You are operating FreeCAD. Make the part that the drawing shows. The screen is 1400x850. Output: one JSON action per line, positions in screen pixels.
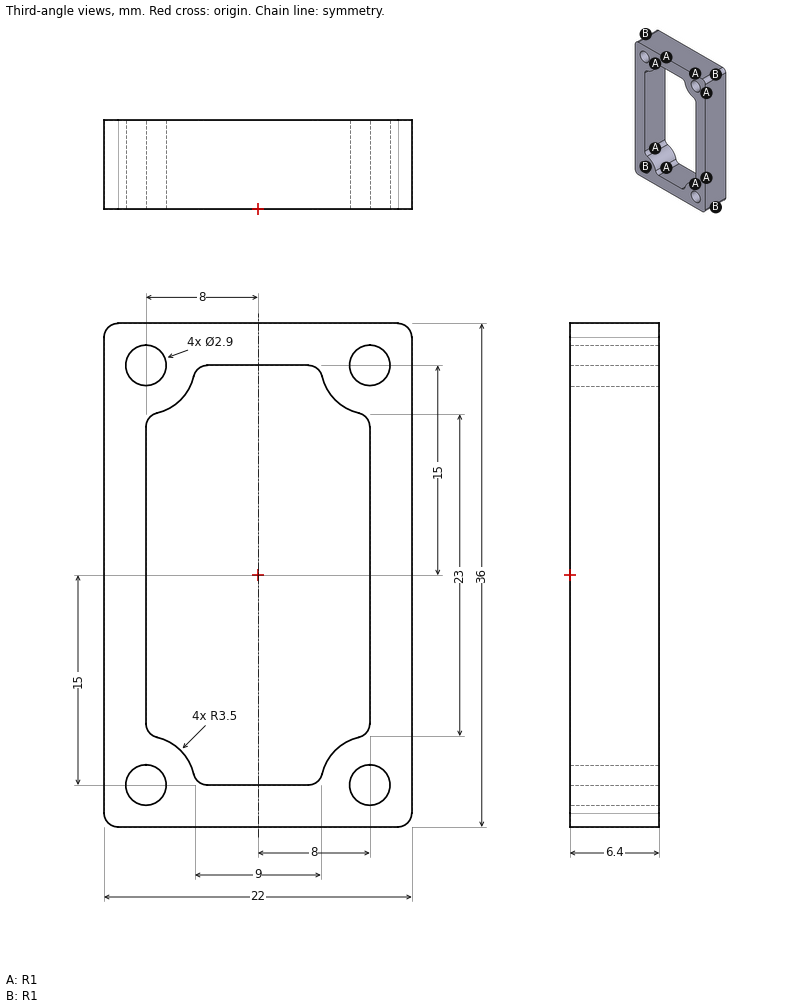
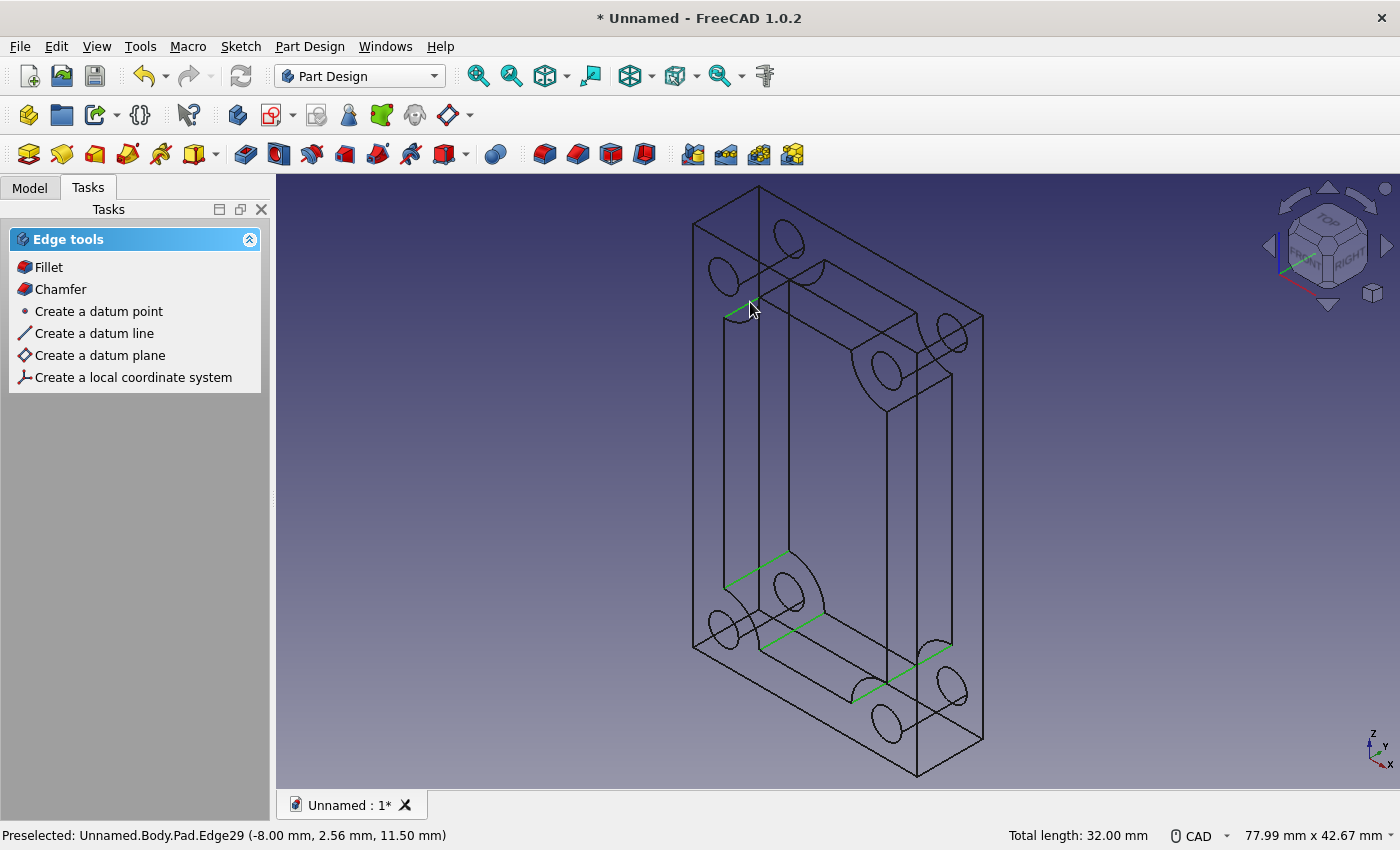
{"action": "left_click", "coordinate": [799, 274], "text": "ctrl"}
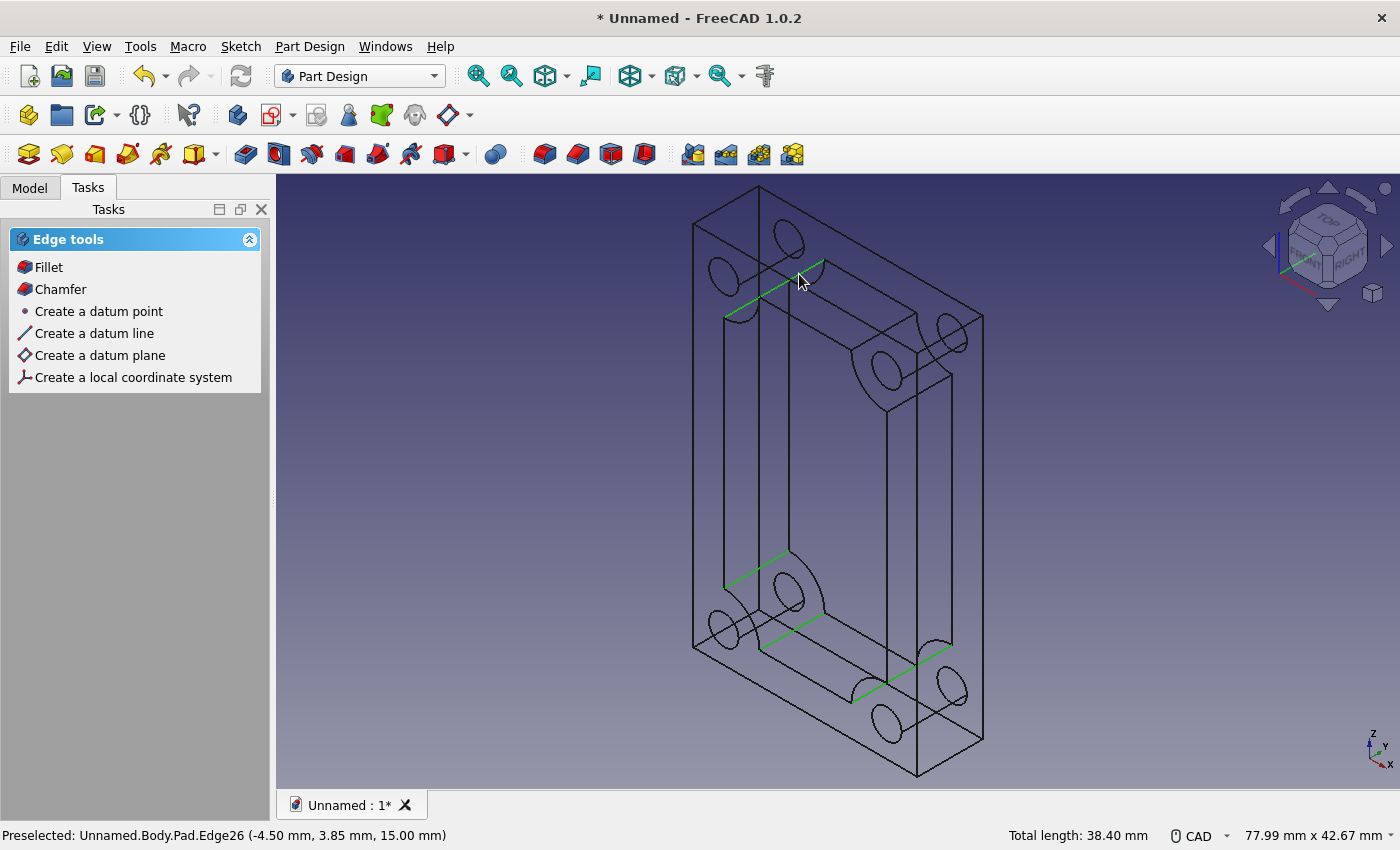
{"action": "left_click", "coordinate": [890, 327], "text": "ctrl"}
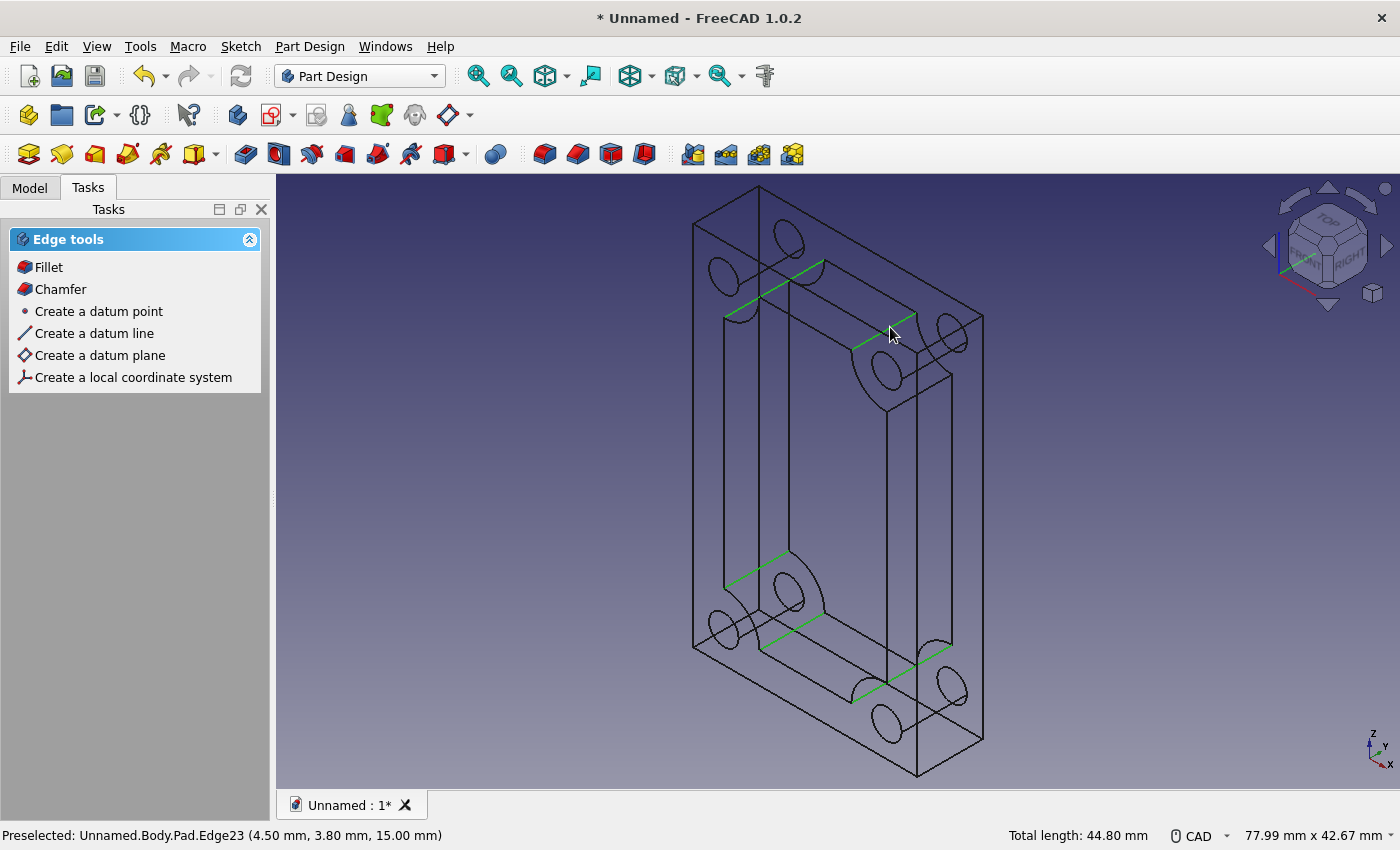
{"action": "left_click", "coordinate": [926, 388], "text": "ctrl"}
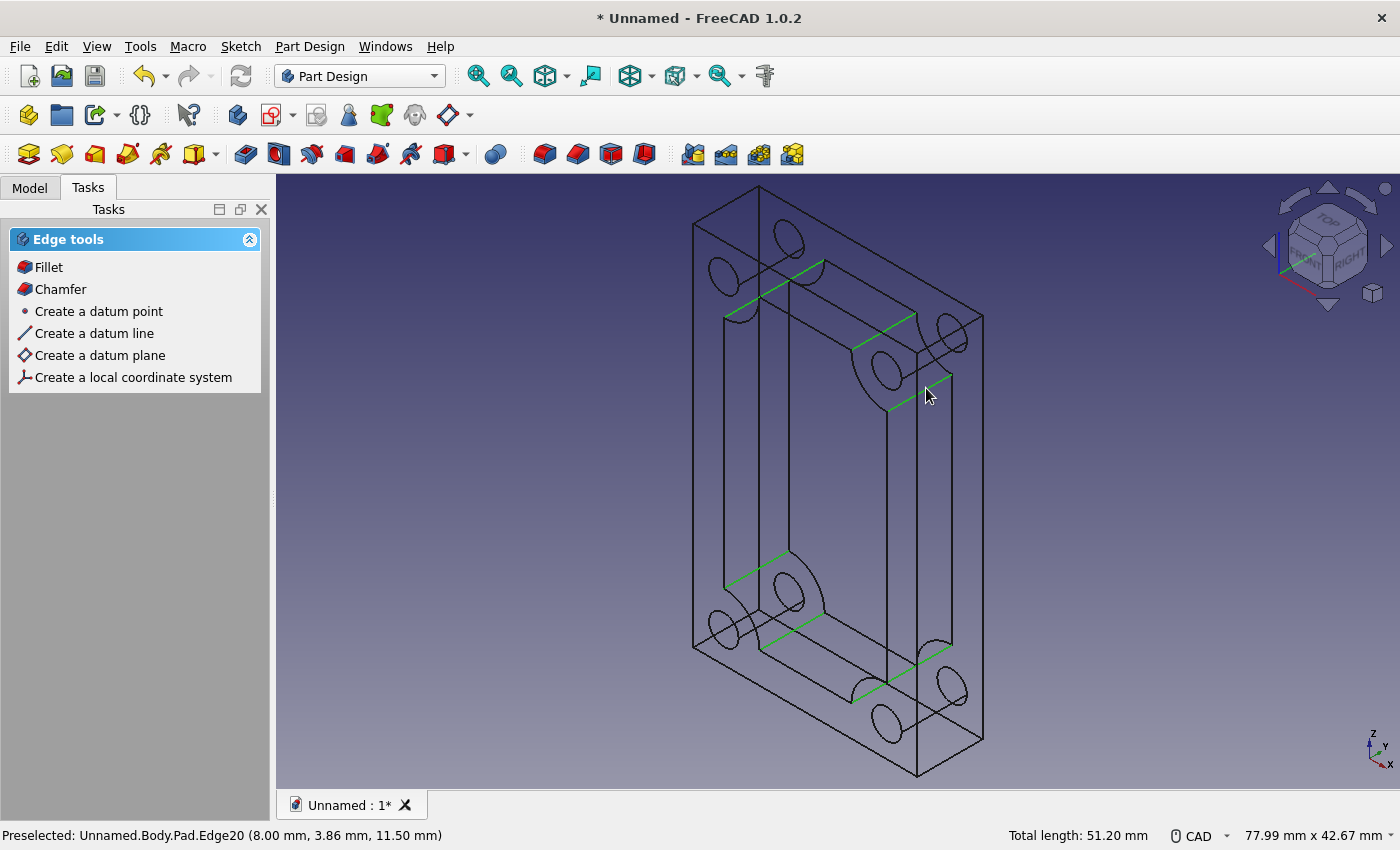
{"action": "key", "text": "v 1"}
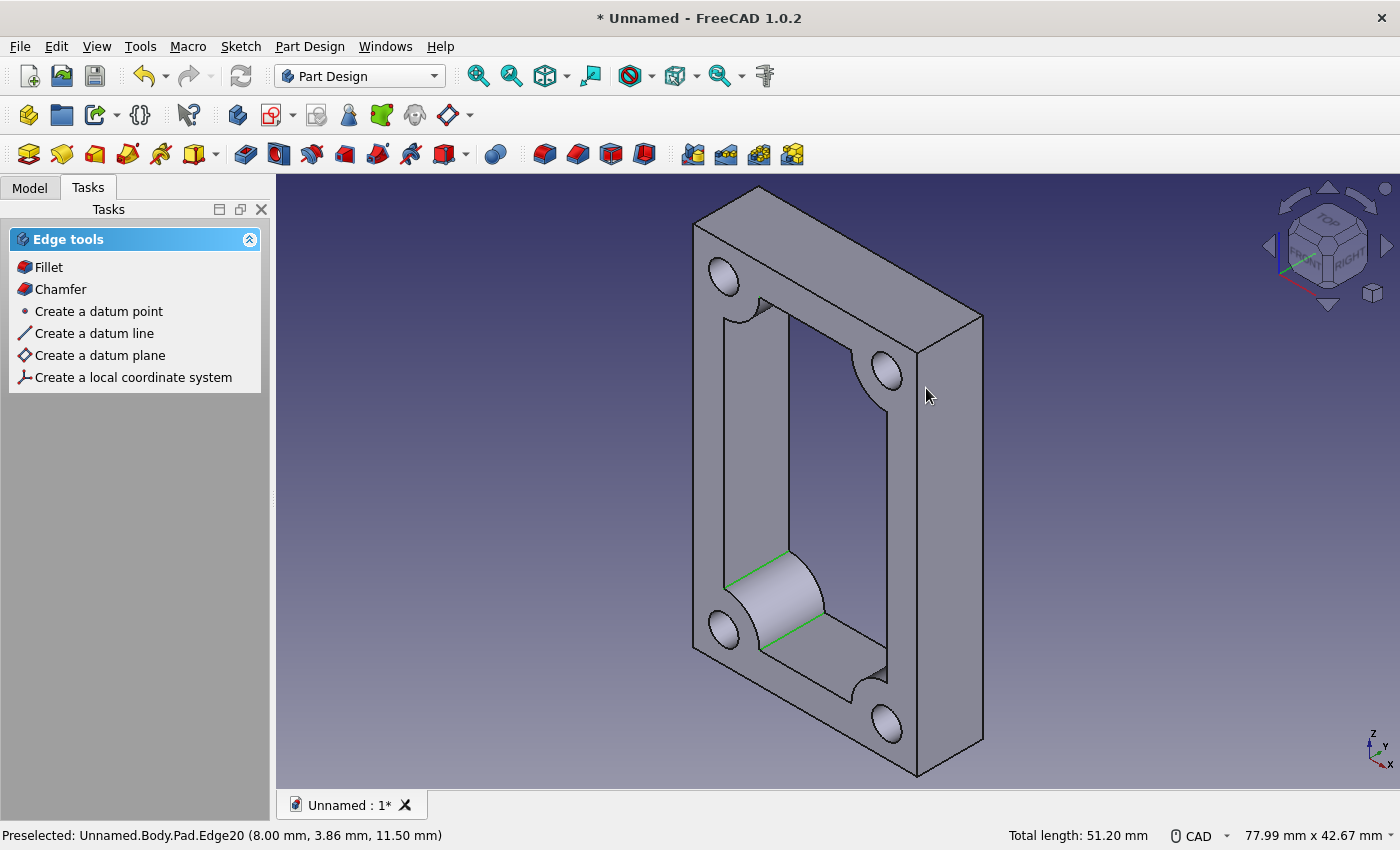
{"action": "left_click", "coordinate": [545, 154]}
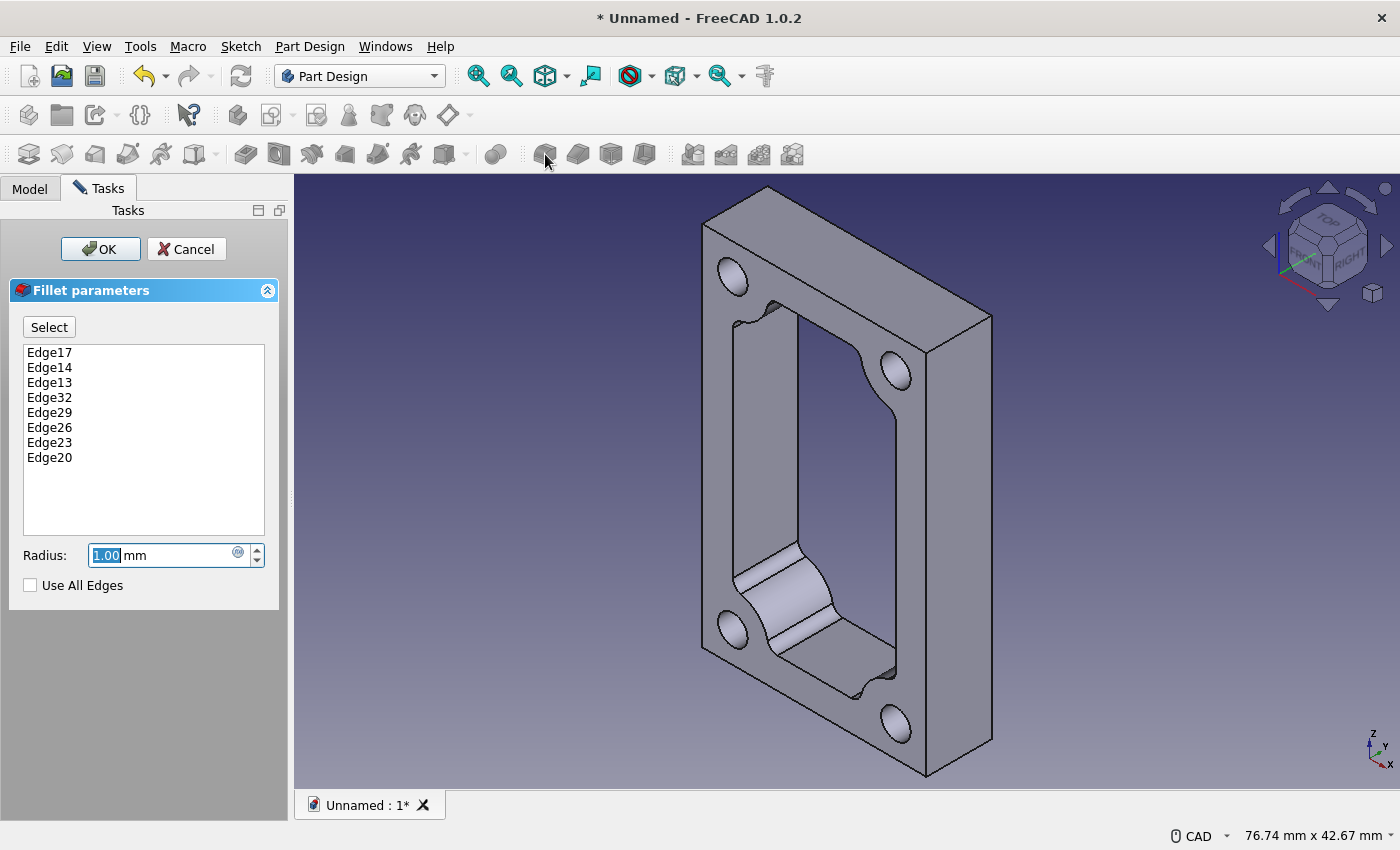
{"action": "type", "text": "1"}
{"action": "key", "text": "Tab"}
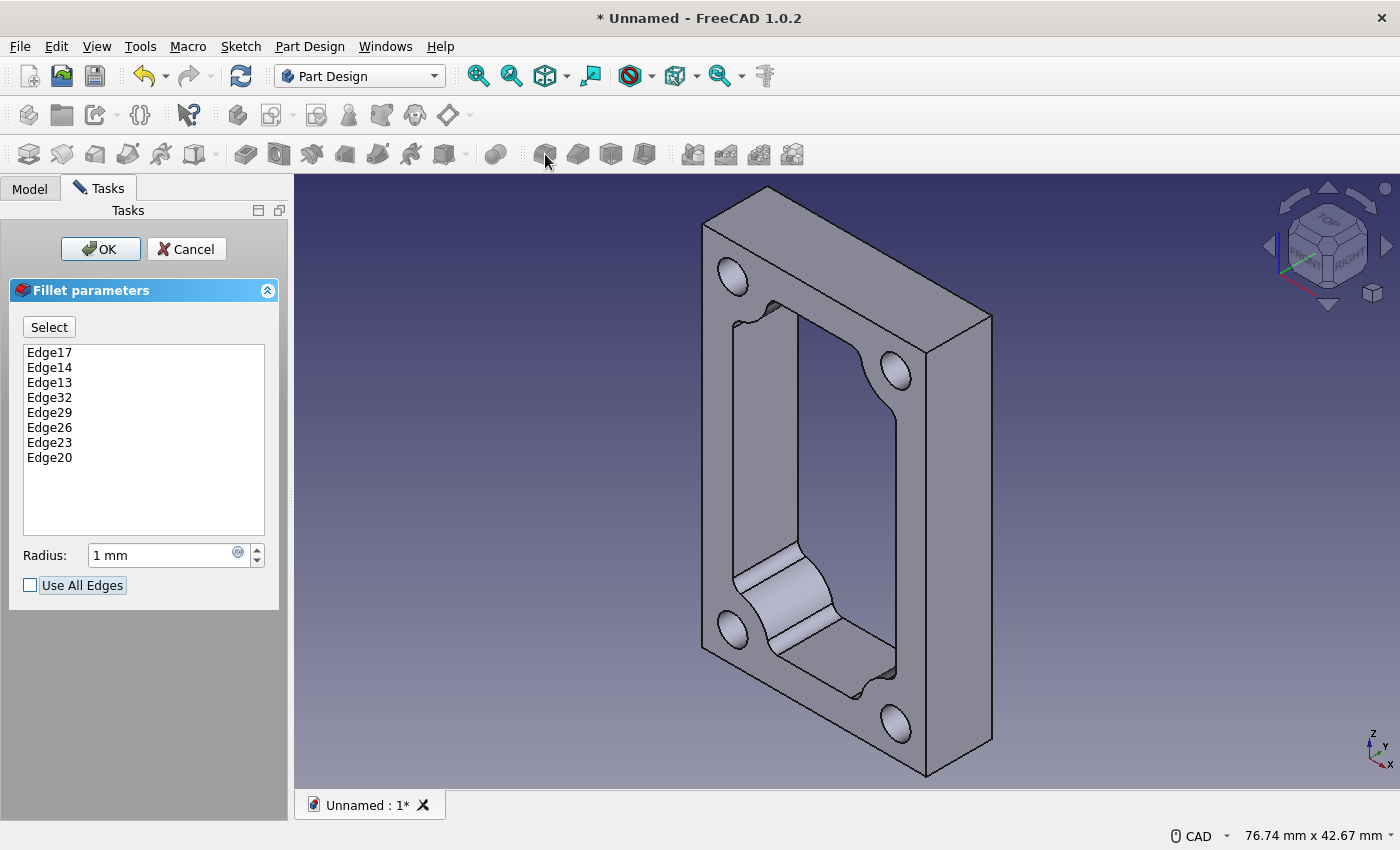
{"action": "left_click", "coordinate": [101, 249]}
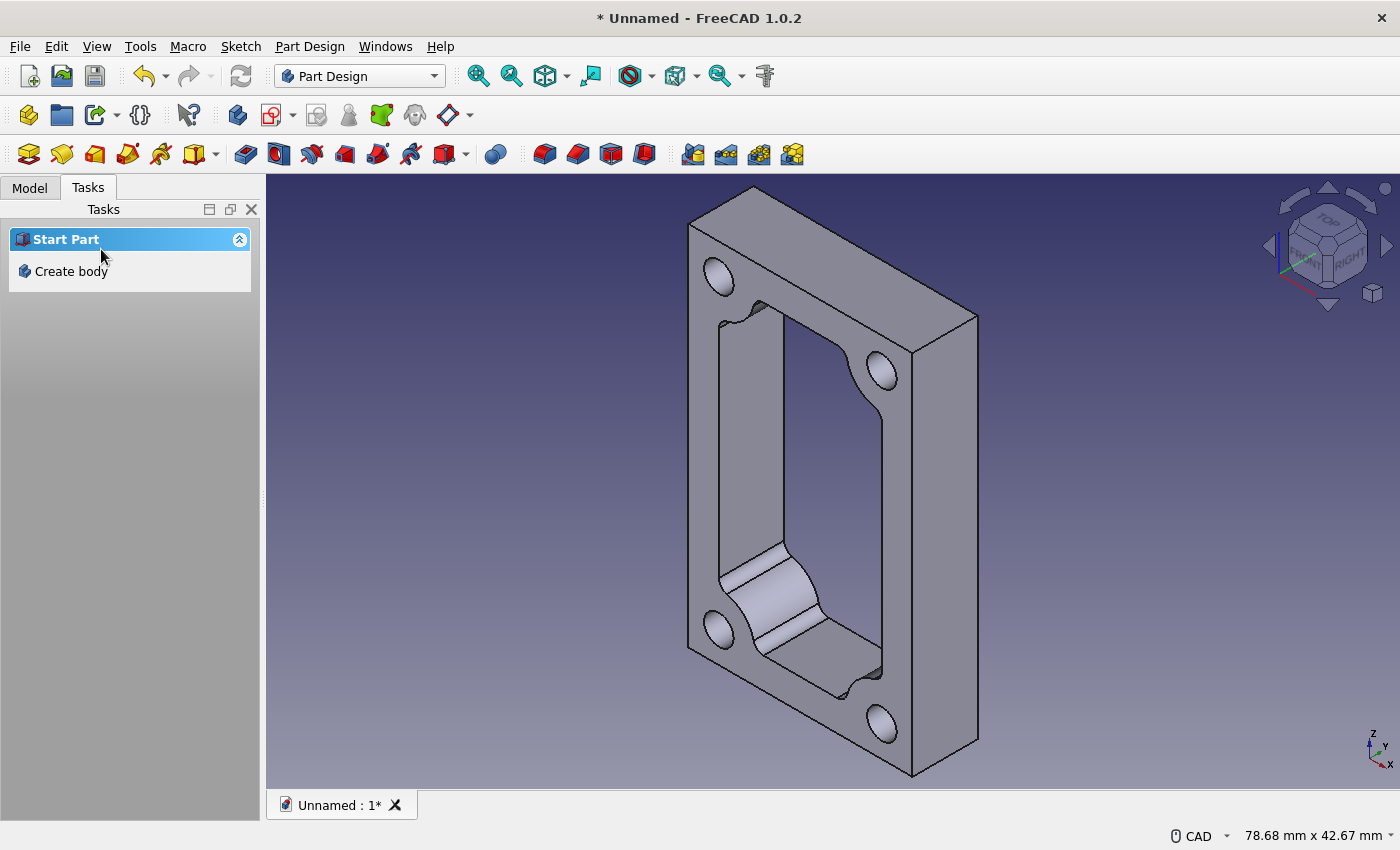
{"action": "left_click", "coordinate": [945, 333]}